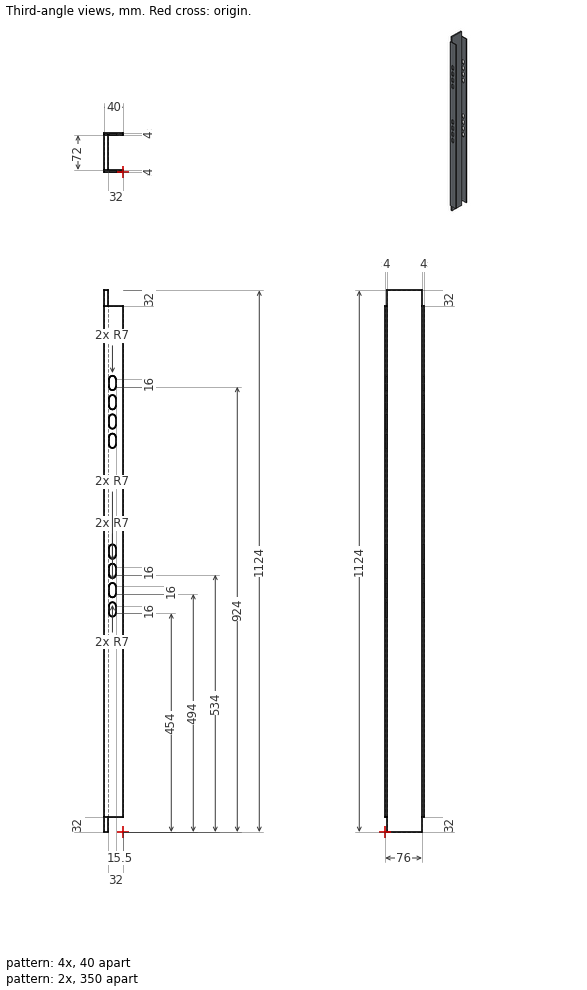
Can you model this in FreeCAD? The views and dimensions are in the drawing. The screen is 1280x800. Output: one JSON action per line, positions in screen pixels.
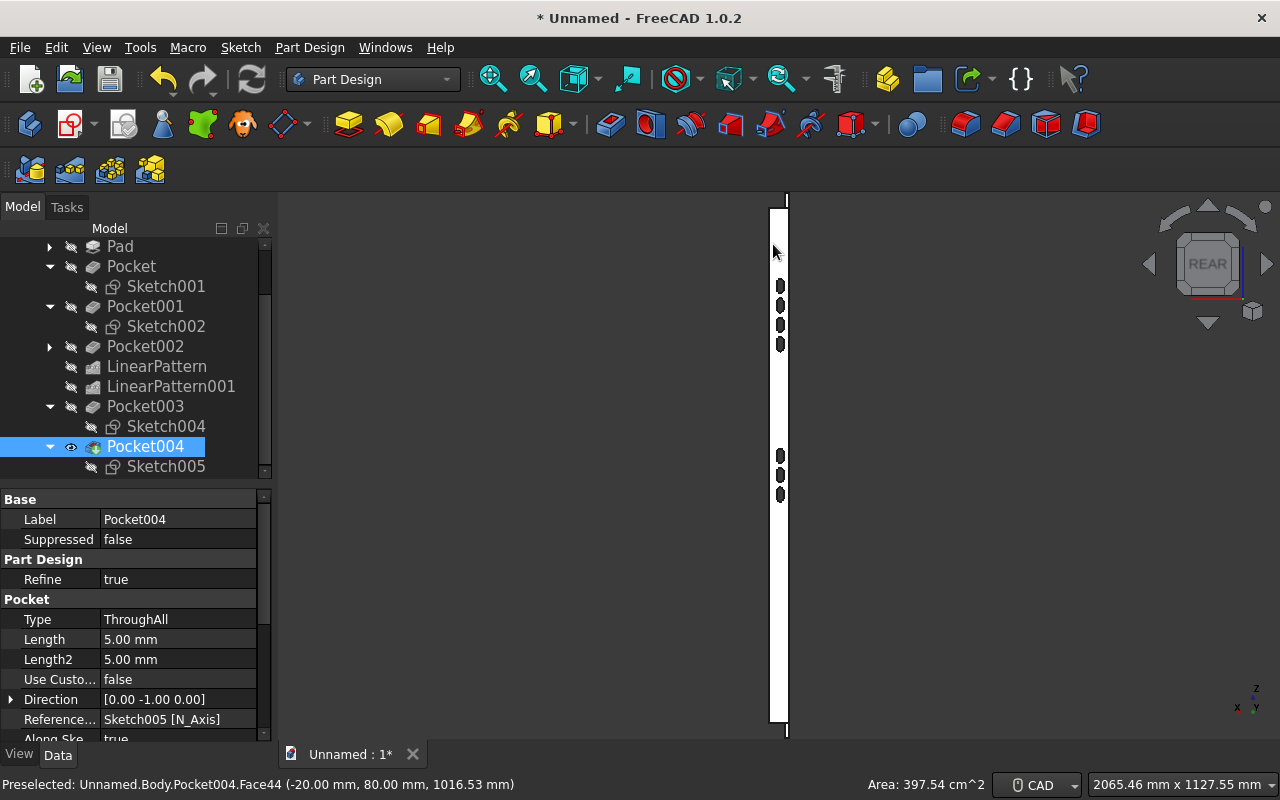
{"action": "left_click", "coordinate": [70, 124]}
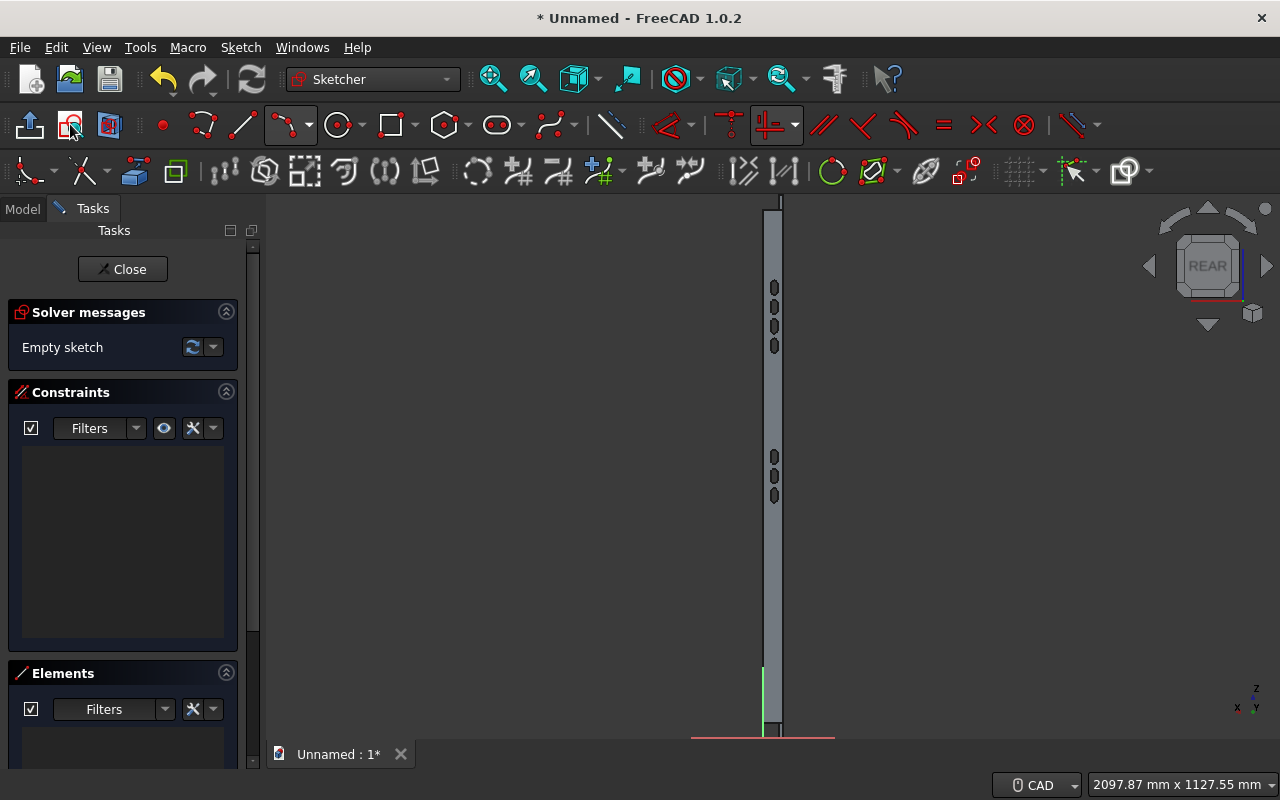
{"action": "scroll", "coordinate": [778, 517], "scroll_direction": "up", "scroll_amount": 15}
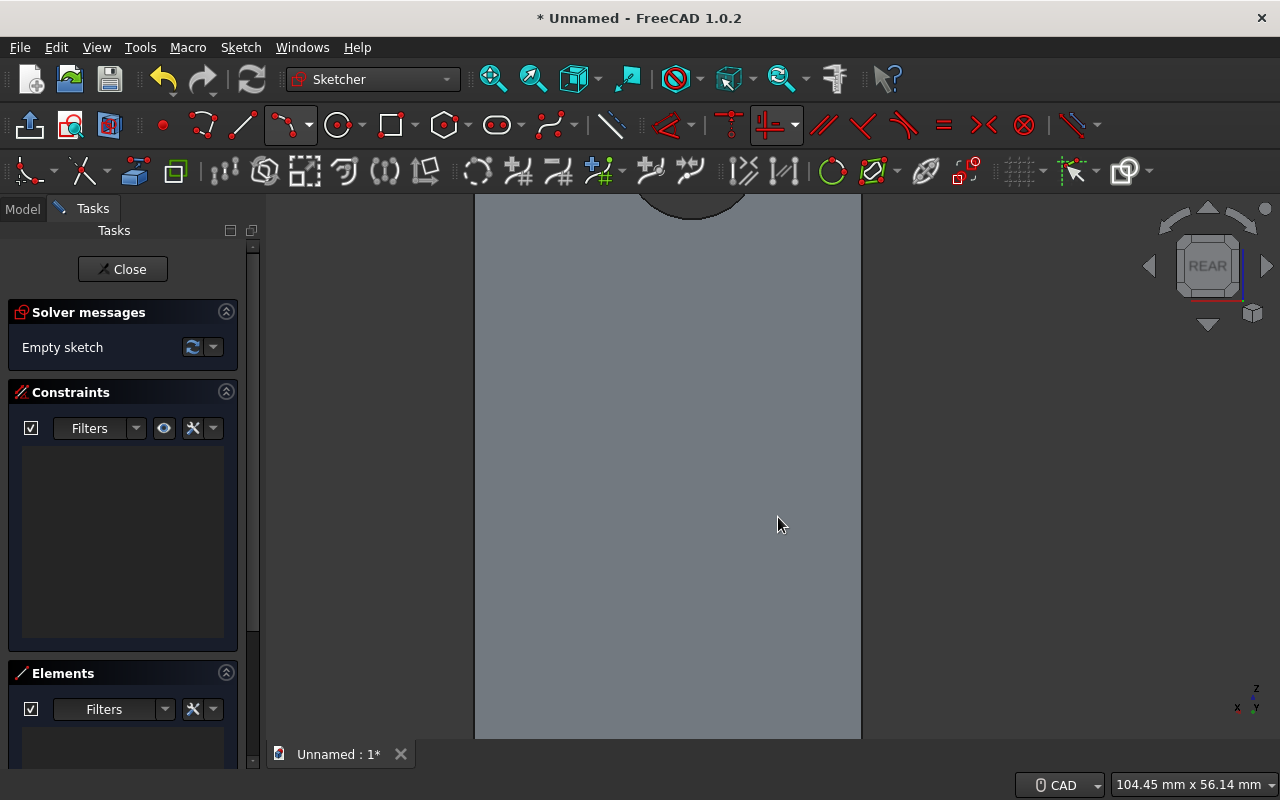
{"action": "key", "text": "g s"}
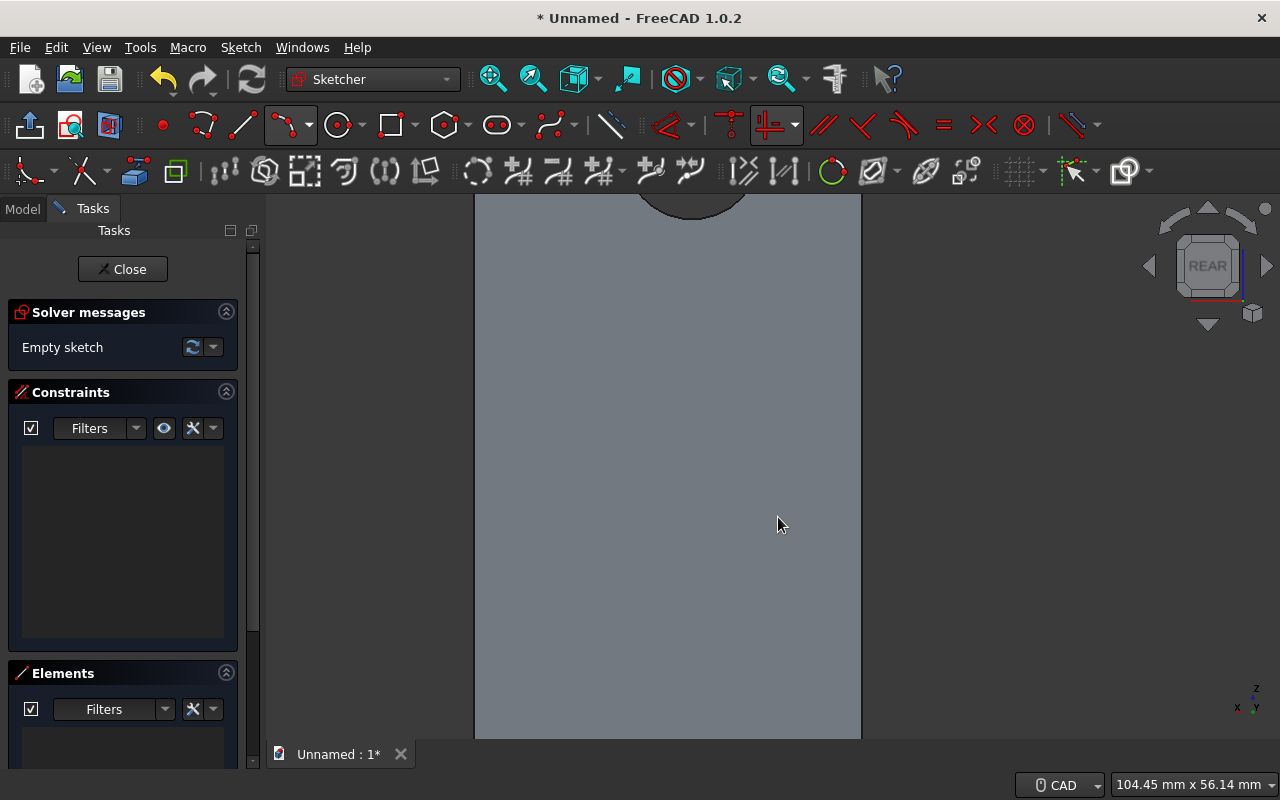
{"action": "left_click", "coordinate": [692, 540]}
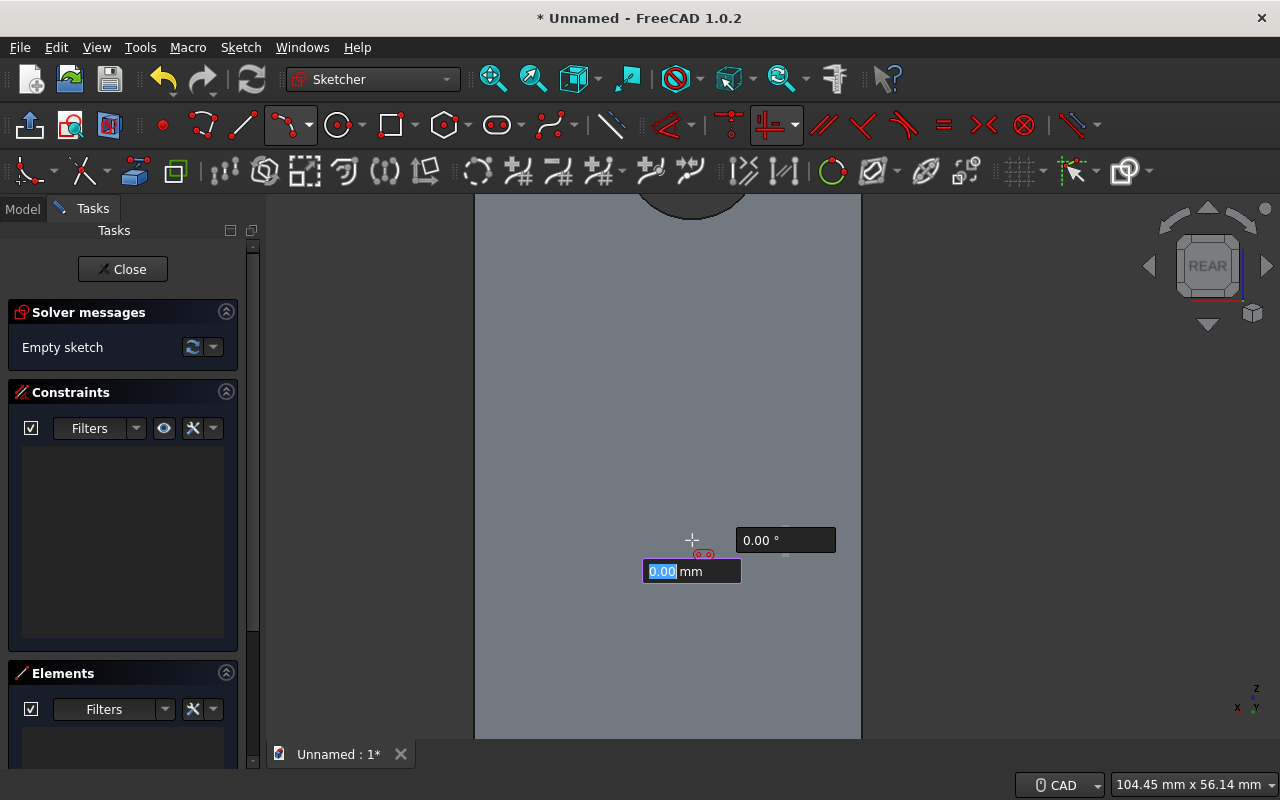
{"action": "left_click", "coordinate": [692, 385]}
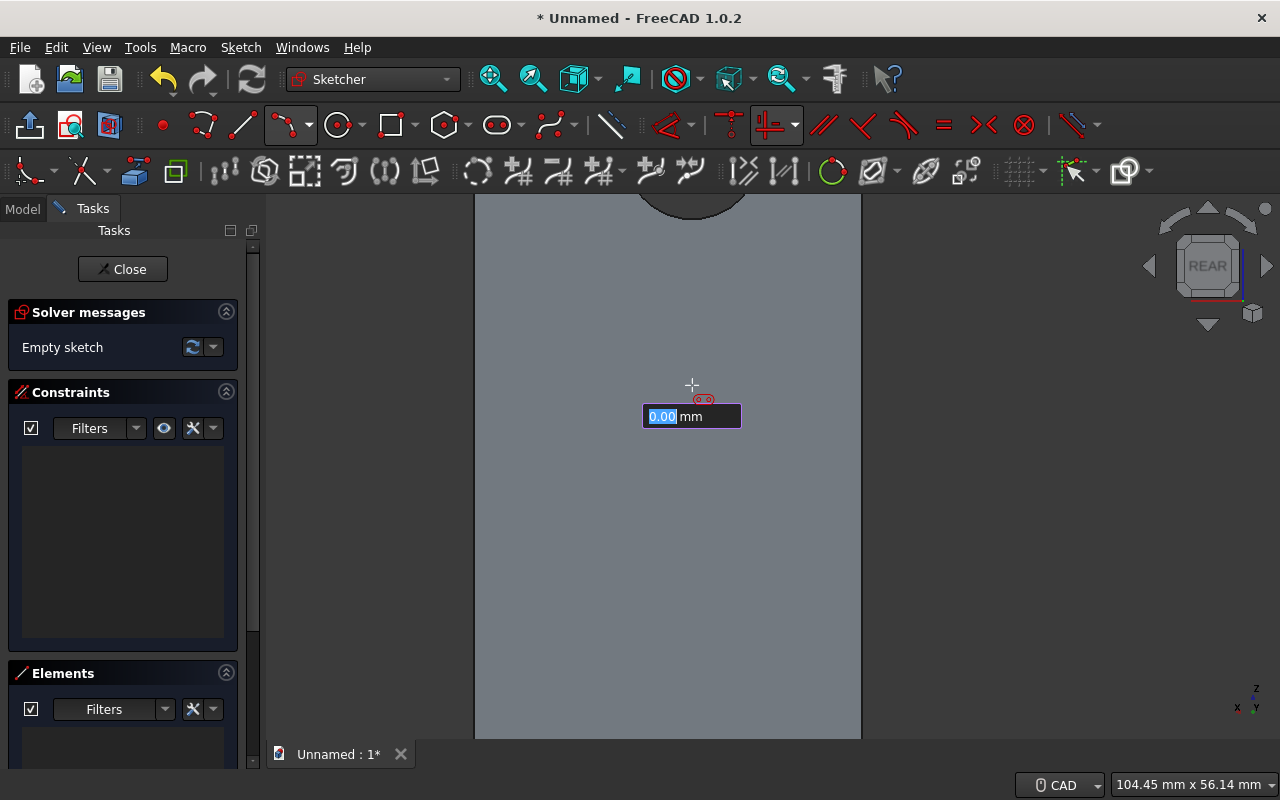
{"action": "left_click", "coordinate": [760, 462]}
{"action": "key", "text": "Escape"}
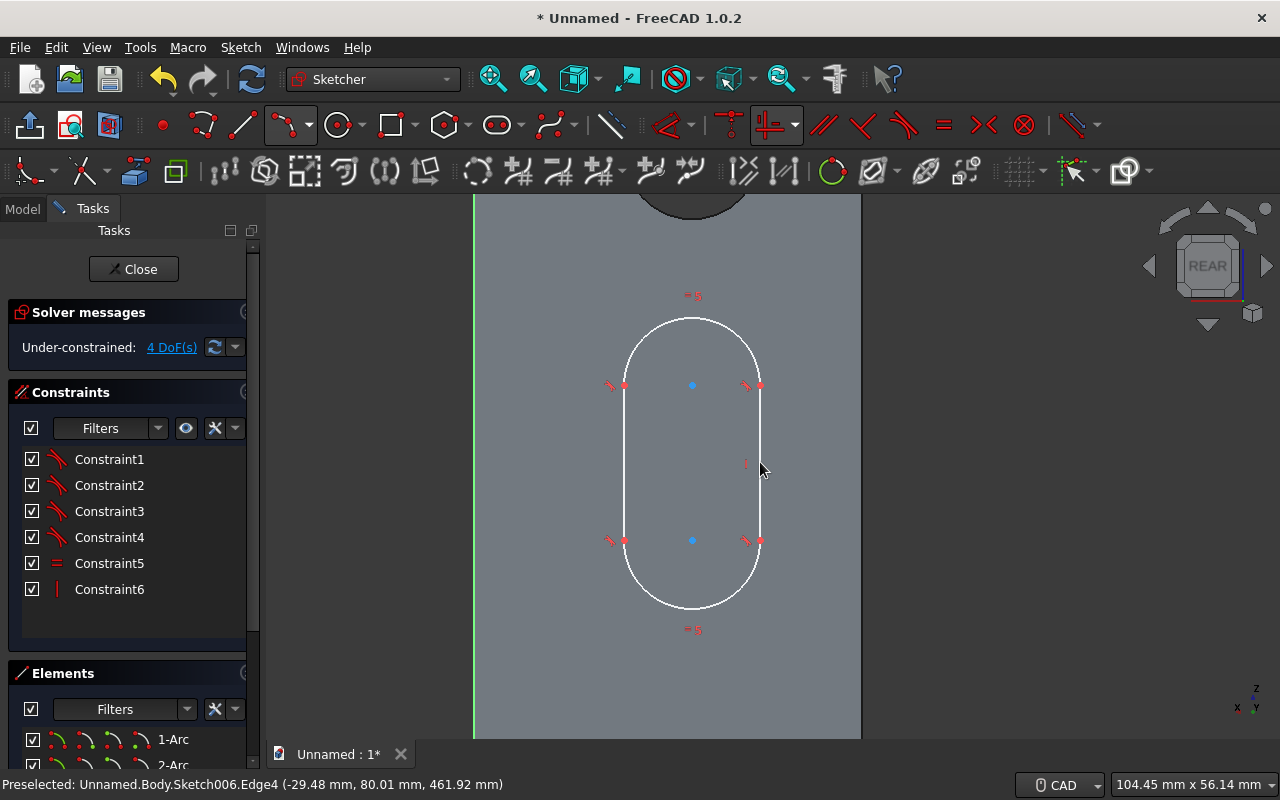
{"action": "left_click", "coordinate": [666, 126]}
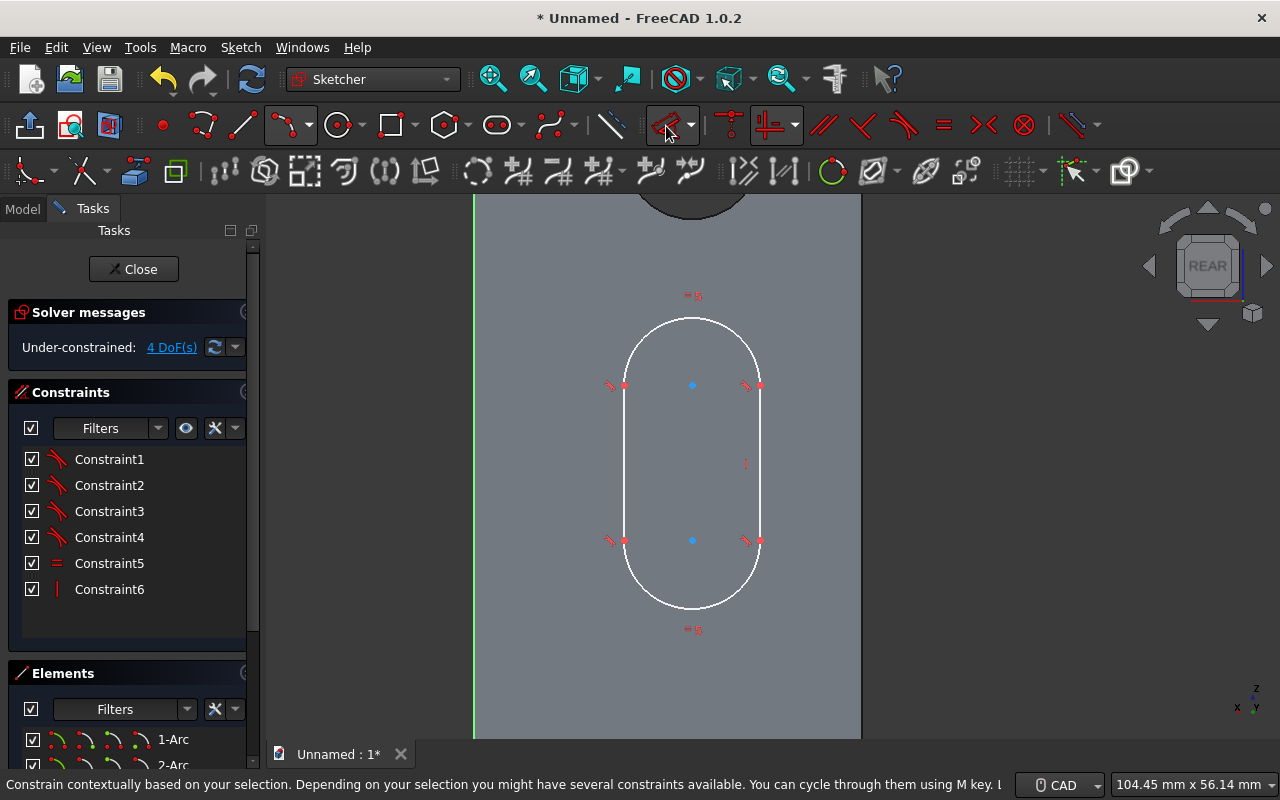
{"action": "left_click", "coordinate": [652, 596]}
{"action": "left_click", "coordinate": [633, 622]}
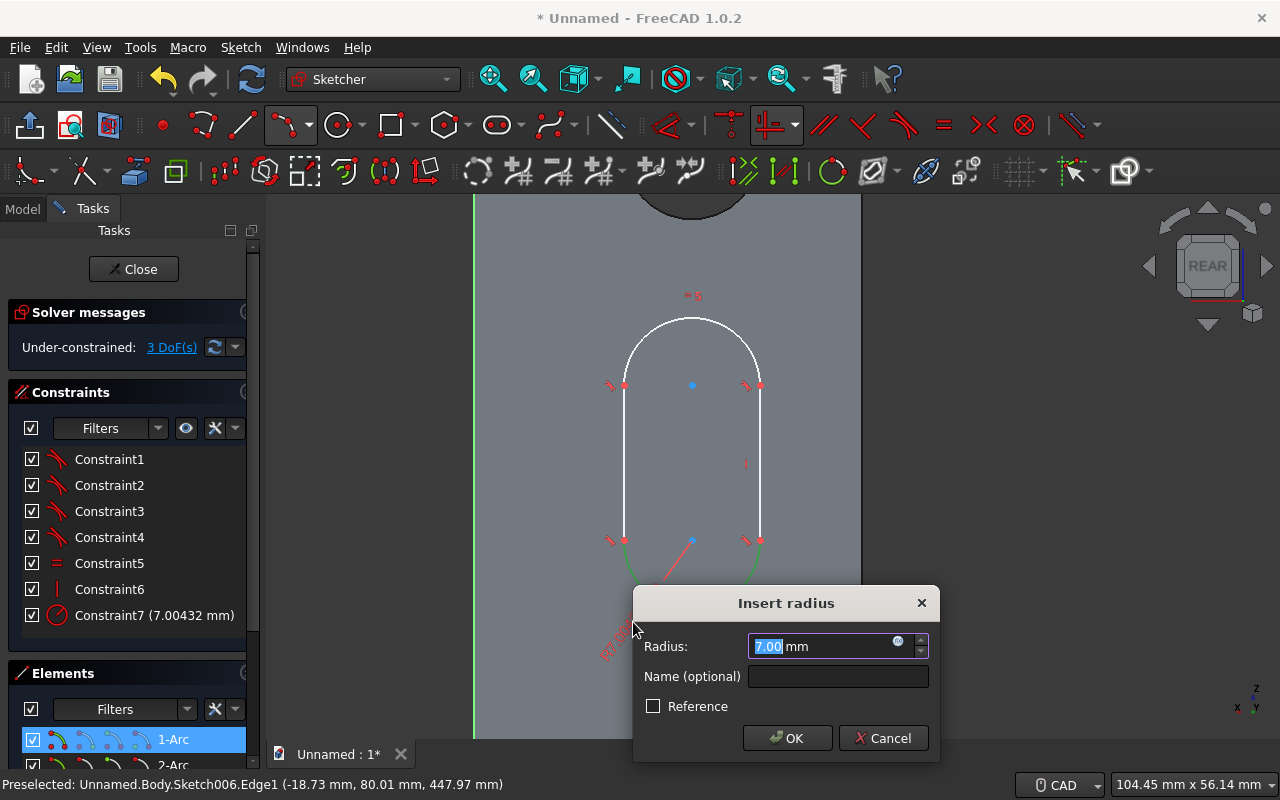
{"action": "type", "text": "7"}
{"action": "key", "text": "Return"}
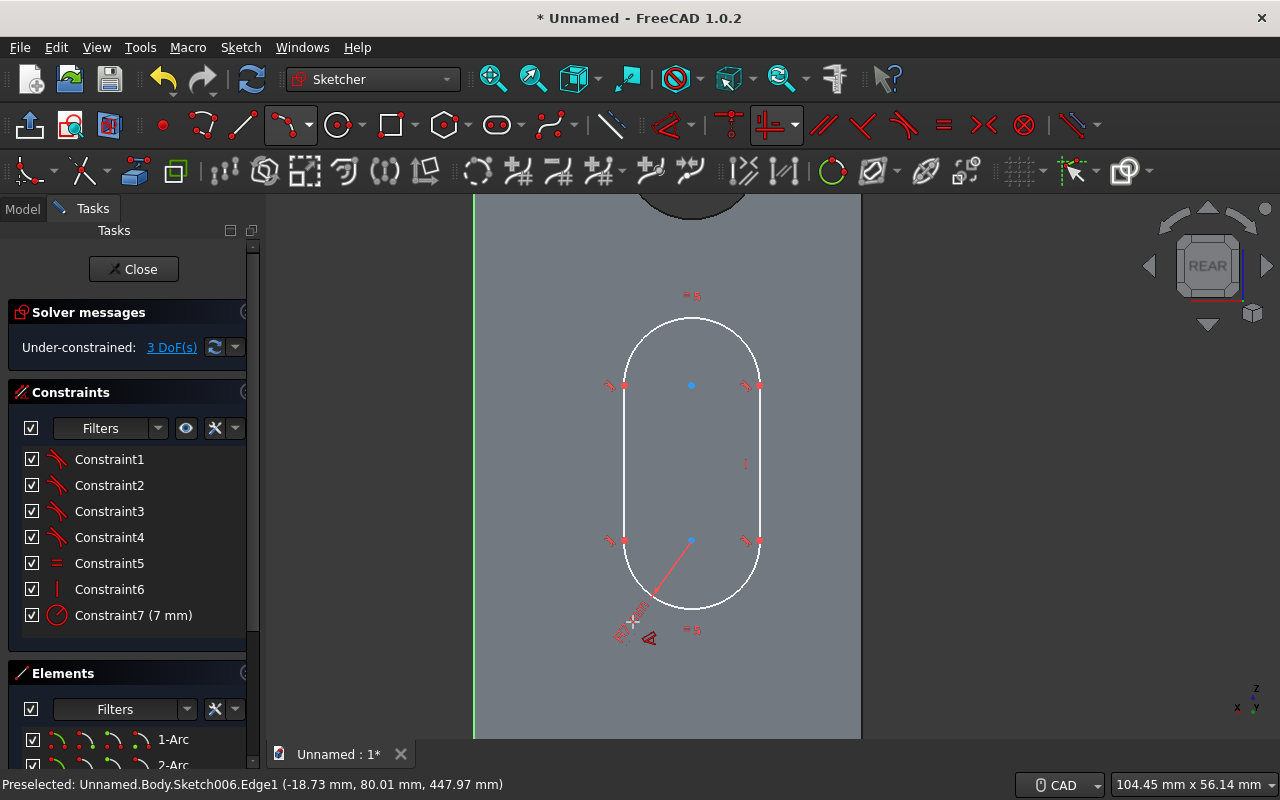
{"action": "left_click", "coordinate": [624, 495]}
{"action": "left_click", "coordinate": [590, 464]}